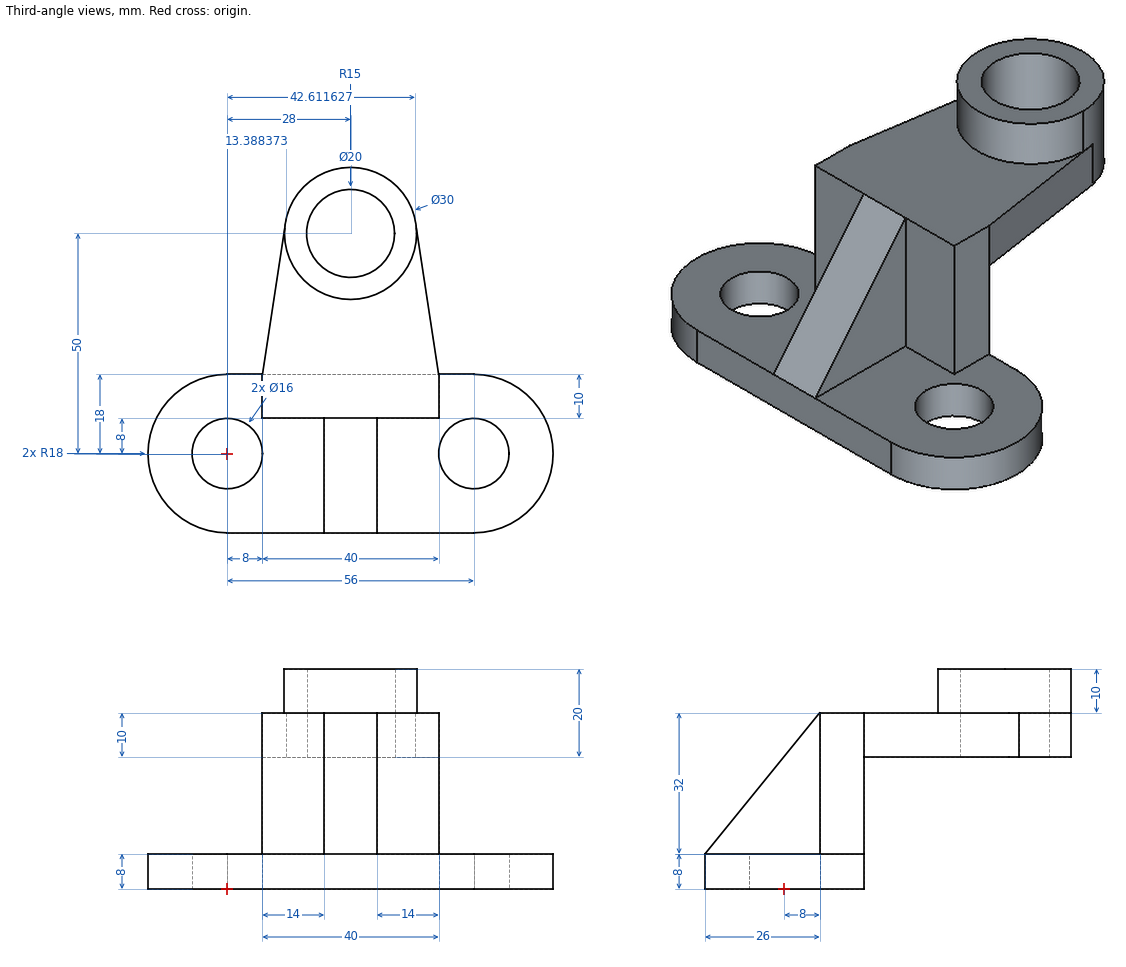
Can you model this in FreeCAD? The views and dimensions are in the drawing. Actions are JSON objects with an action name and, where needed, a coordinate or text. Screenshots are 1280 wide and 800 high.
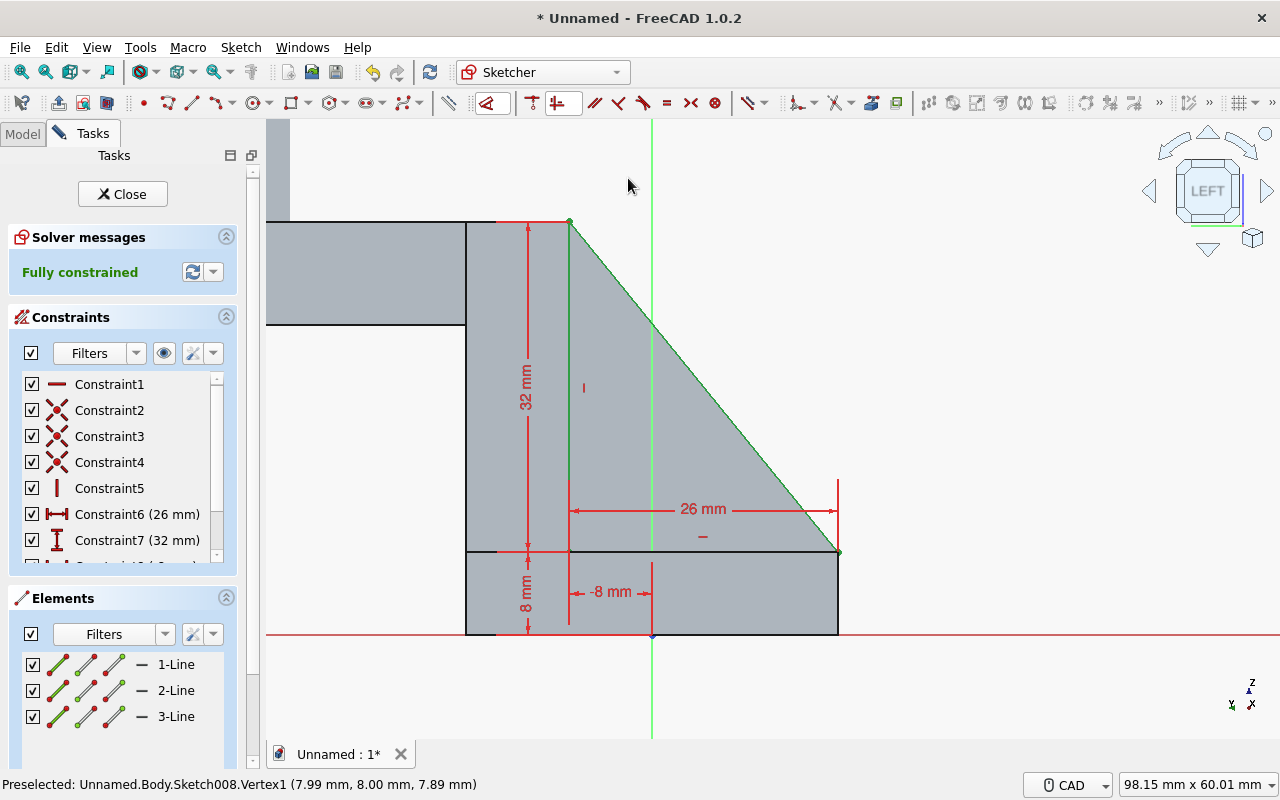
{"action": "left_click", "coordinate": [123, 194]}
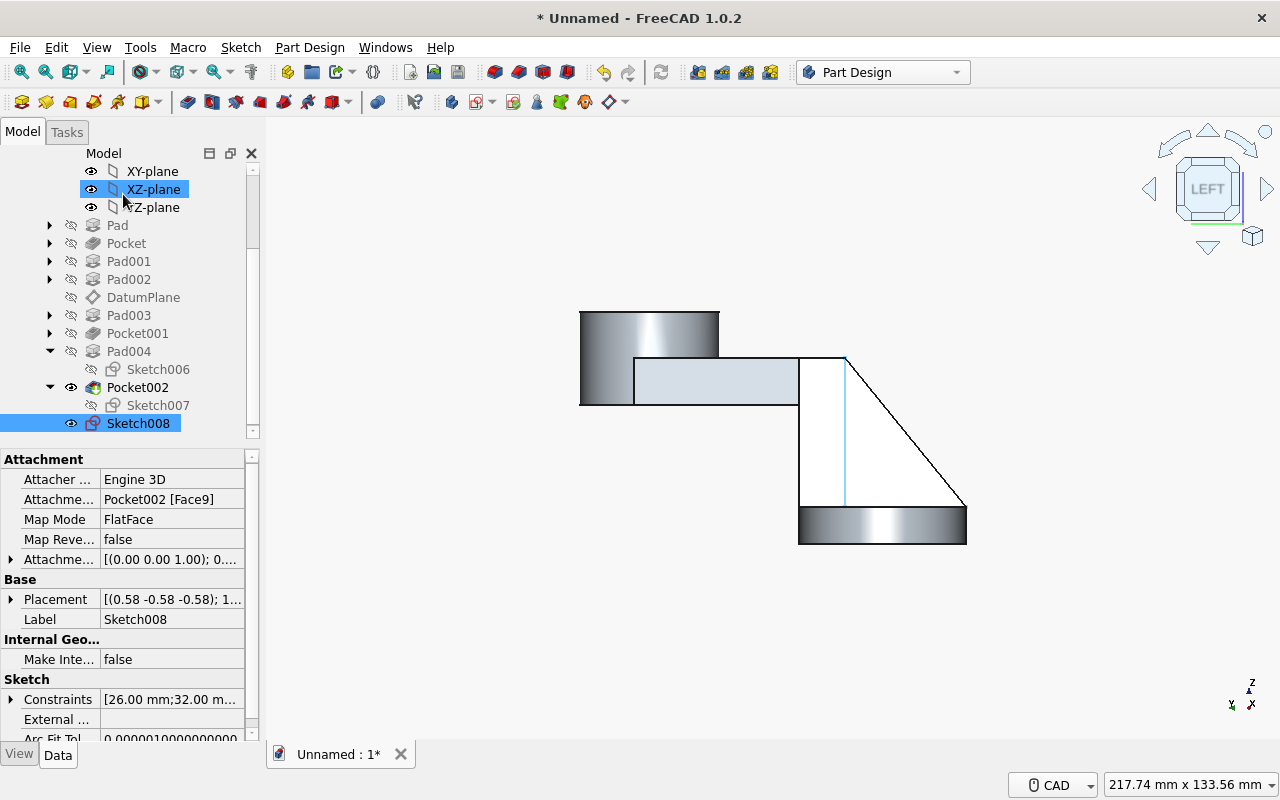
{"action": "left_click", "coordinate": [188, 102]}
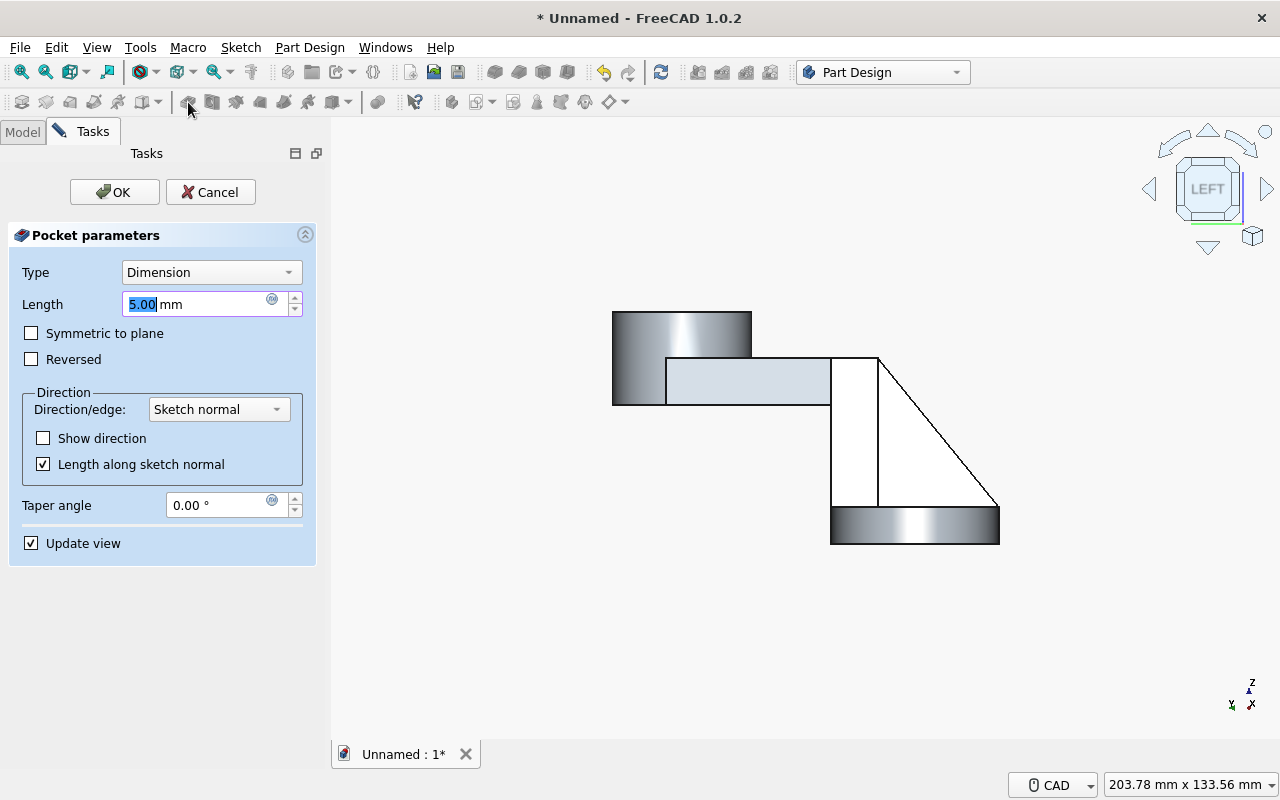
{"action": "type", "text": "14"}
{"action": "key", "text": "Tab"}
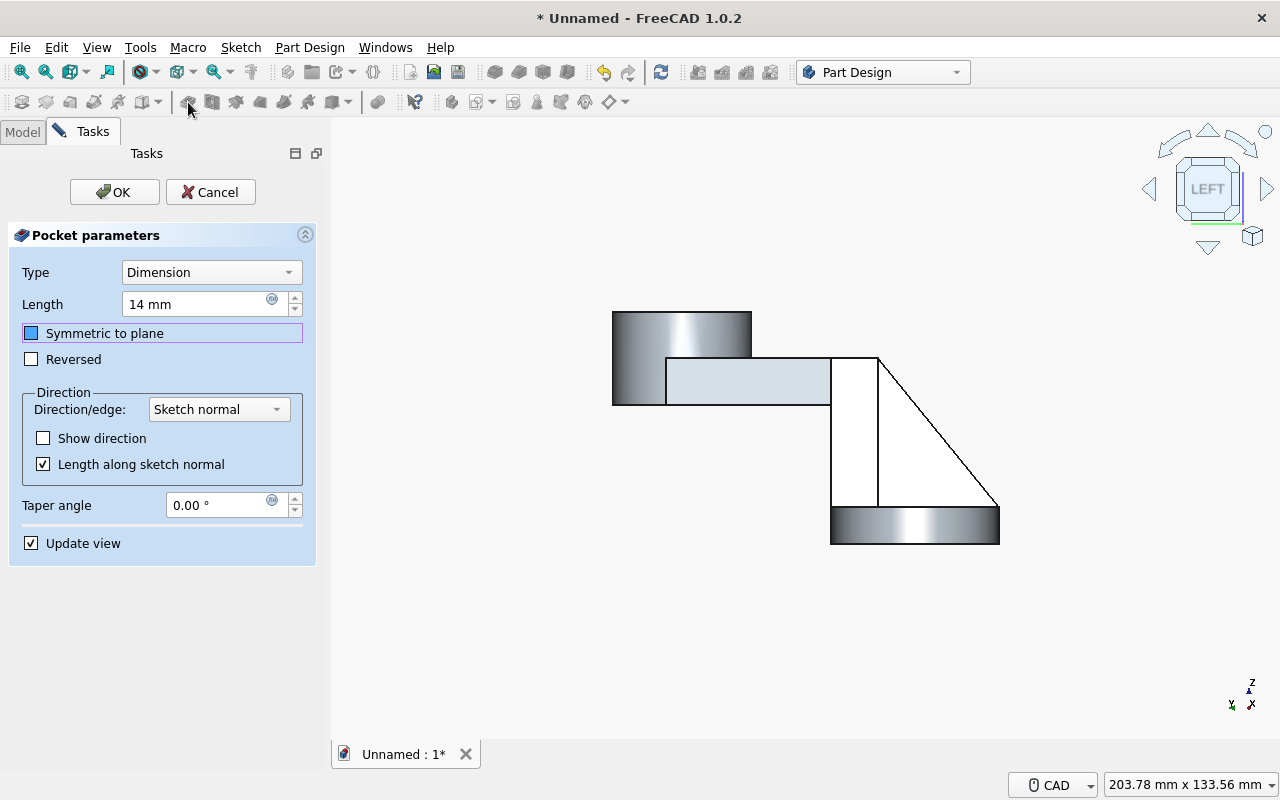
{"action": "left_click", "coordinate": [115, 192]}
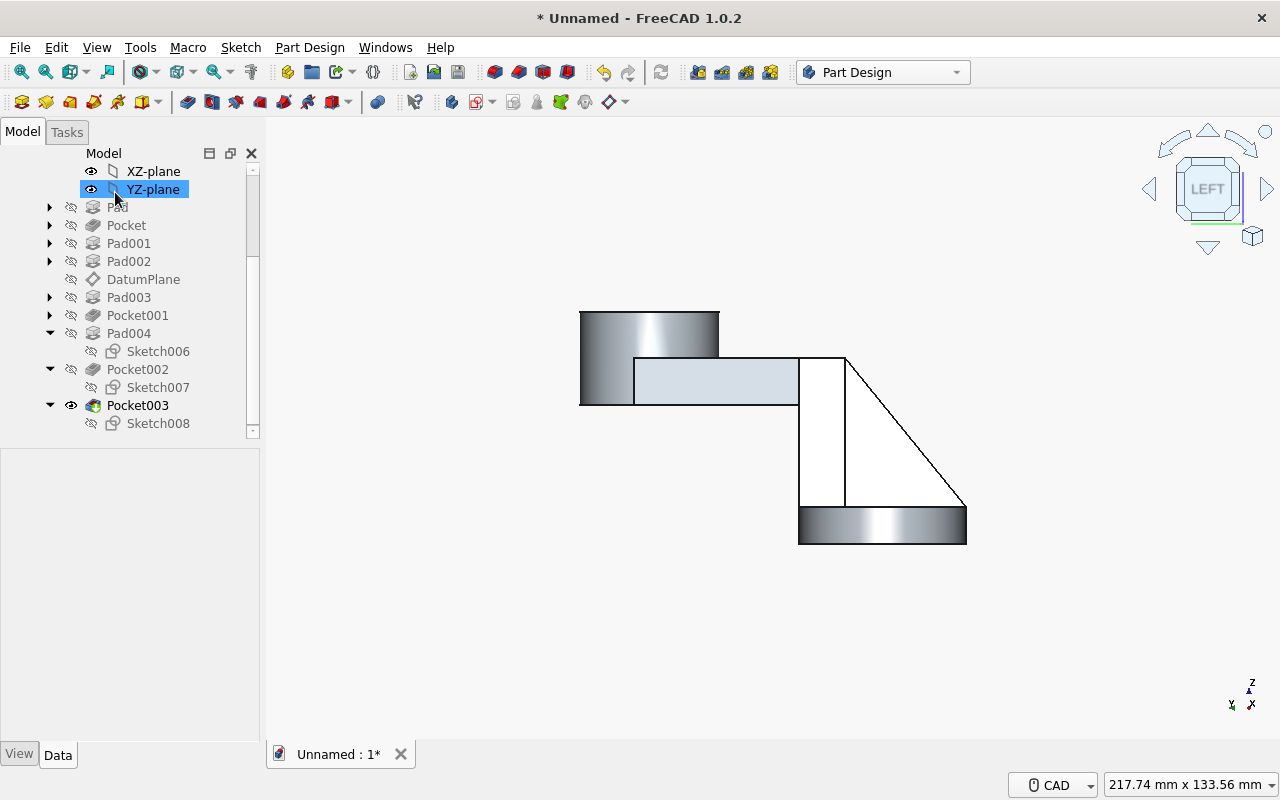
{"action": "key", "text": "0"}